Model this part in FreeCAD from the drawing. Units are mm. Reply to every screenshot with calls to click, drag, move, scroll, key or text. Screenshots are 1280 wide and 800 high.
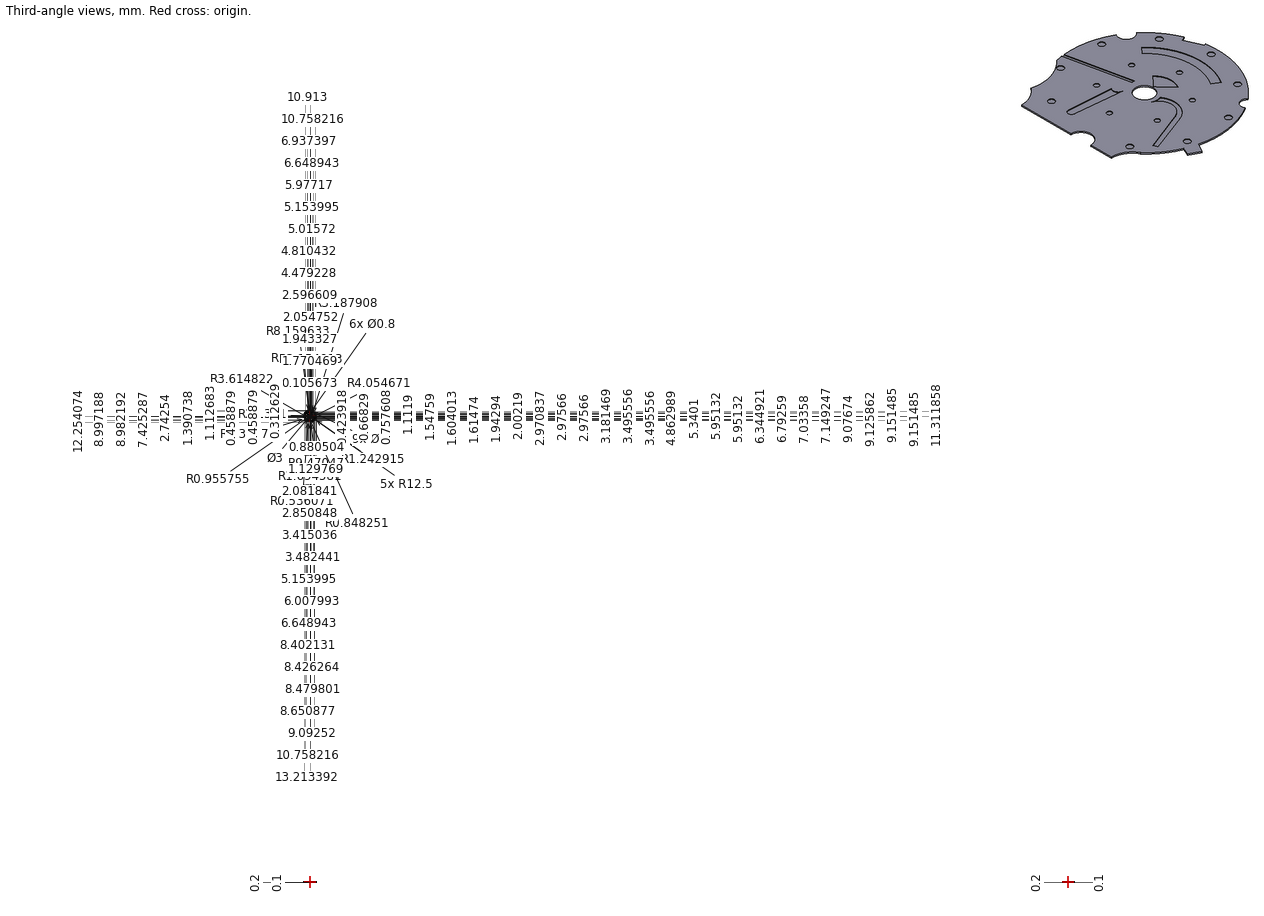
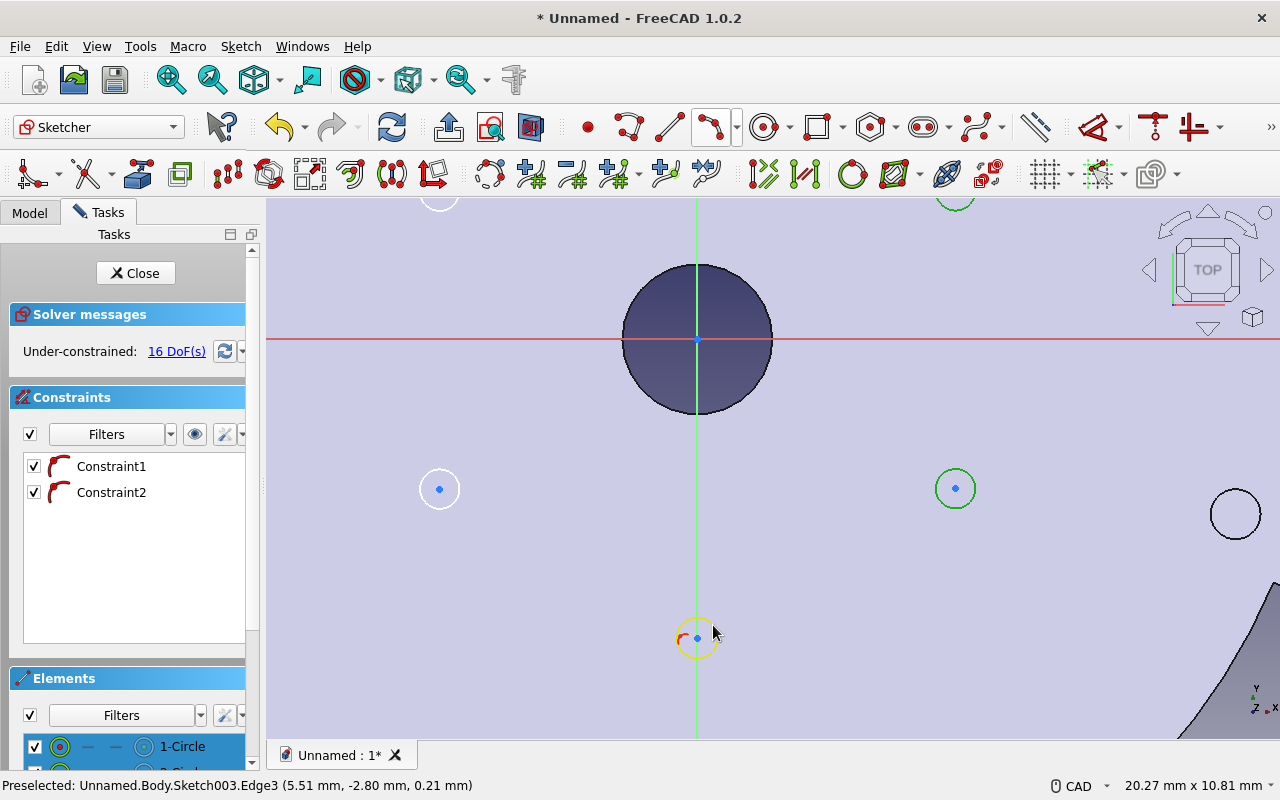
click(712, 624)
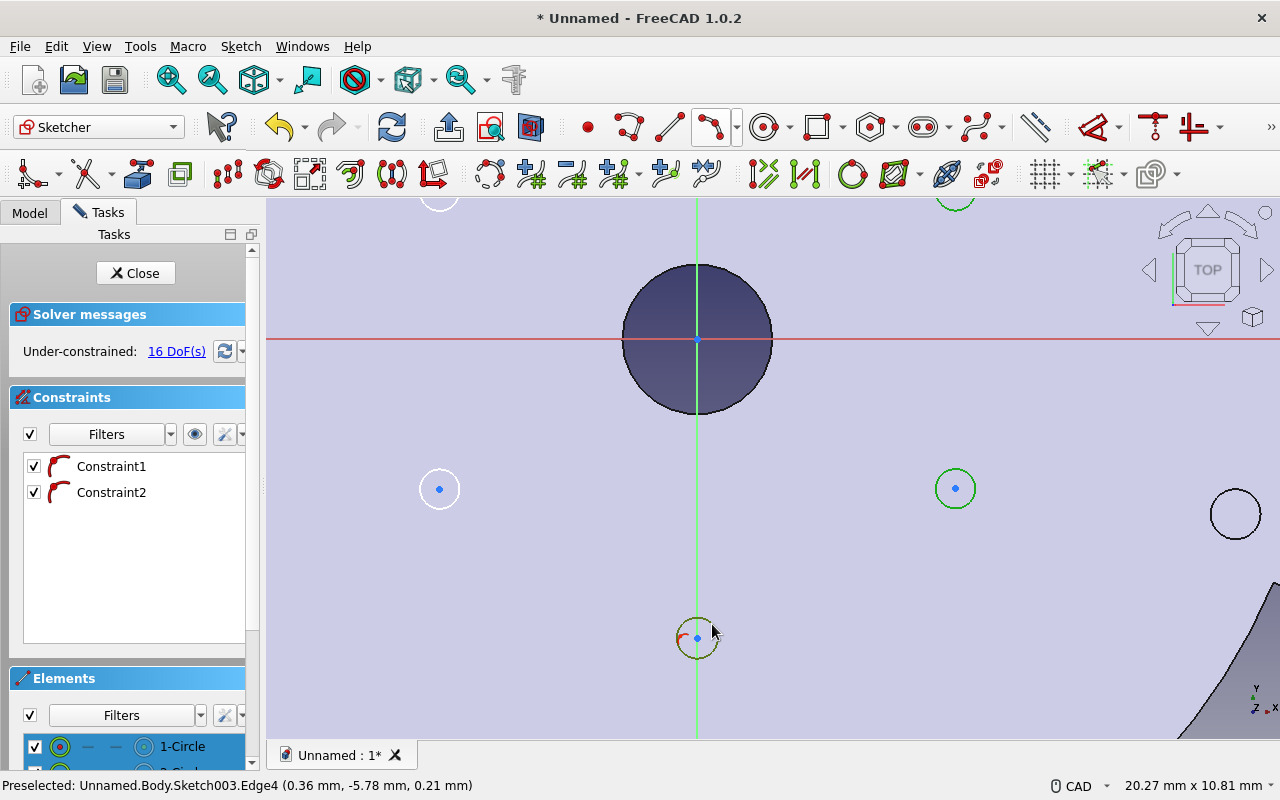
click(454, 475)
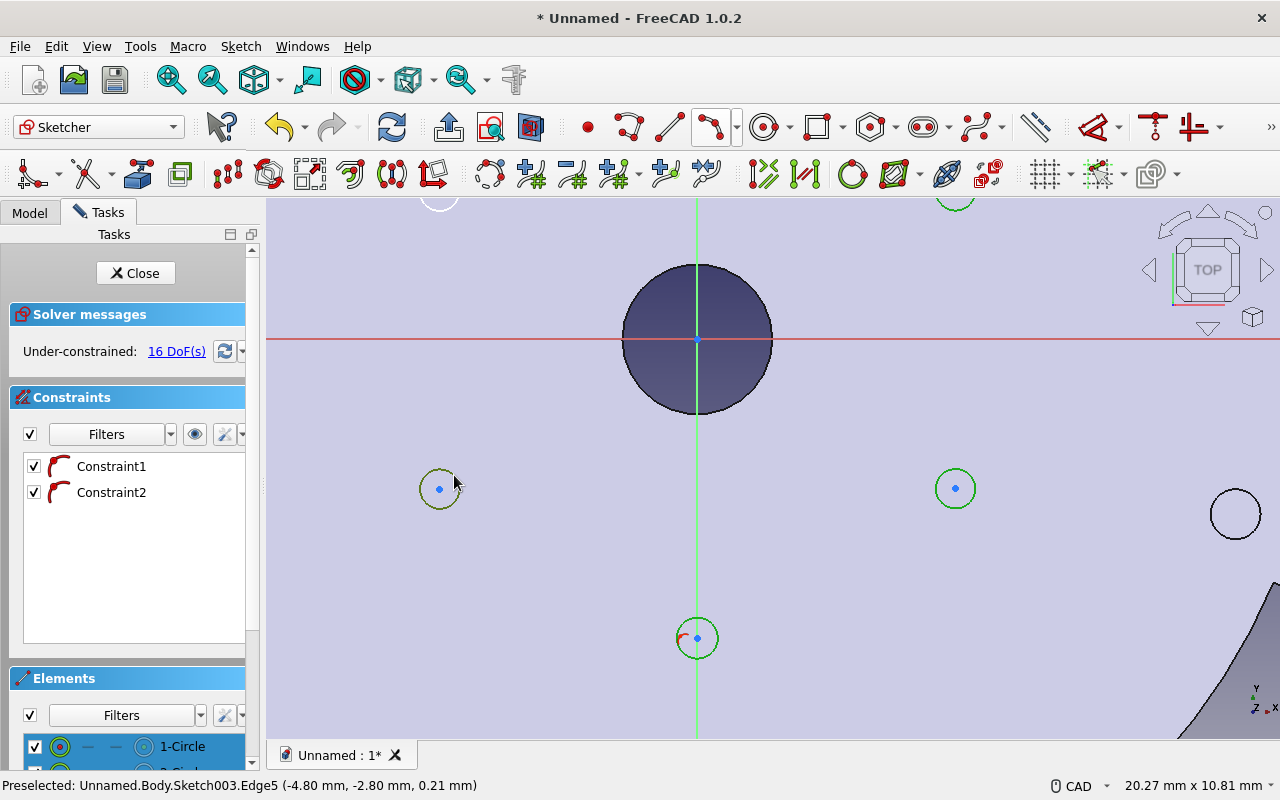
scroll(713, 626, down, 3)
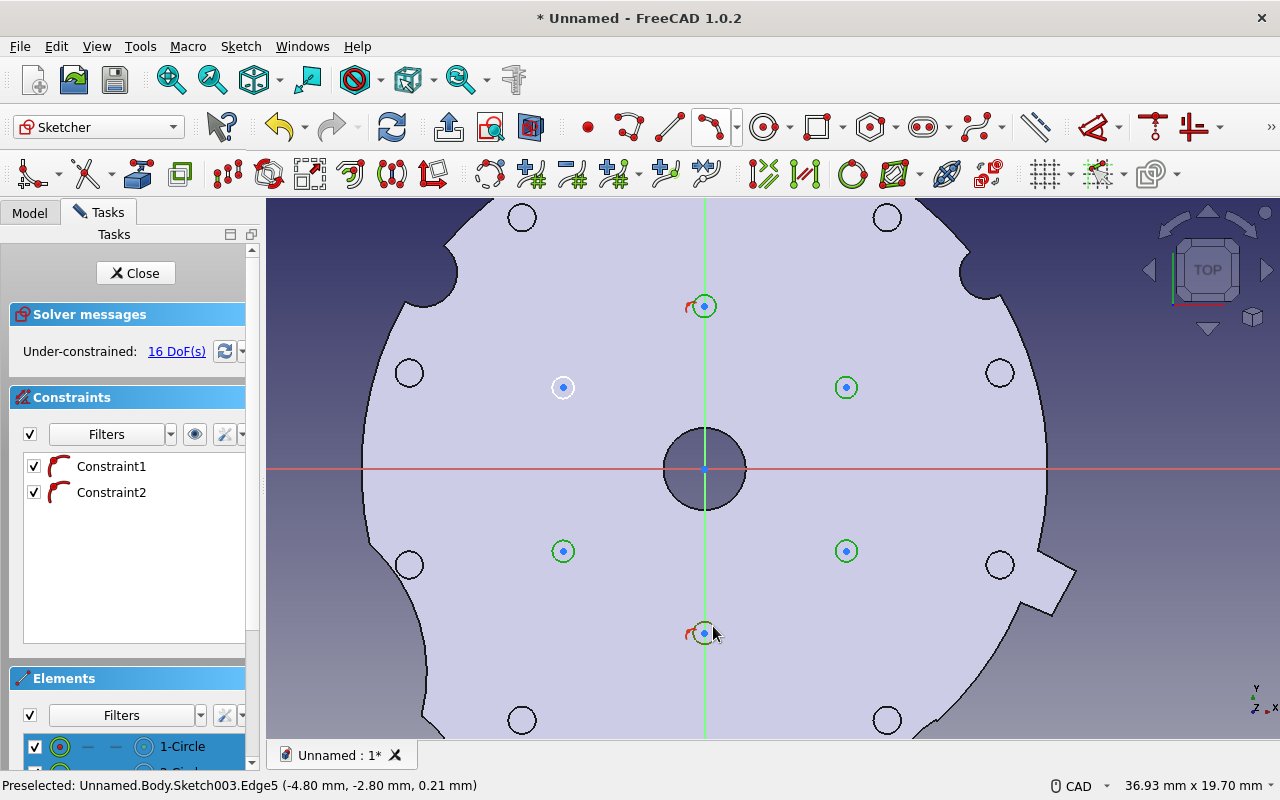
scroll(571, 380, up, 2)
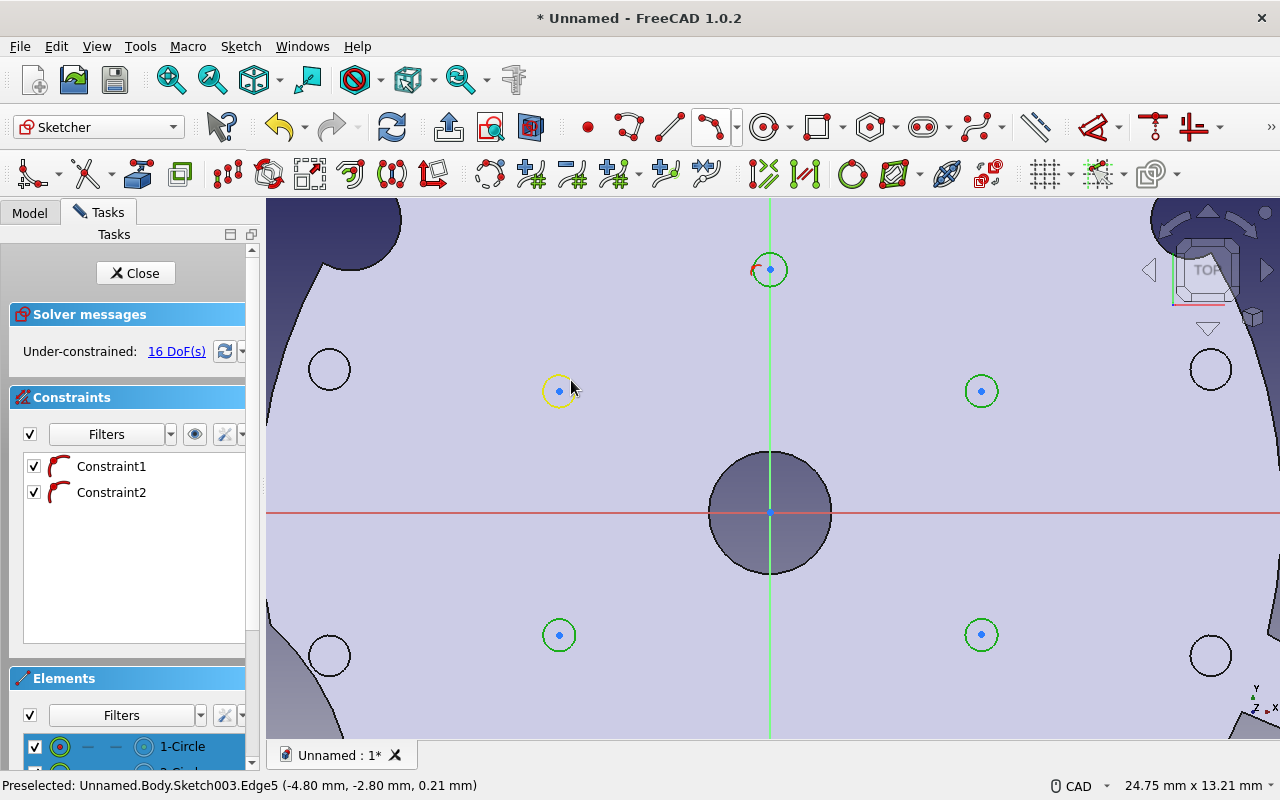
click(571, 380)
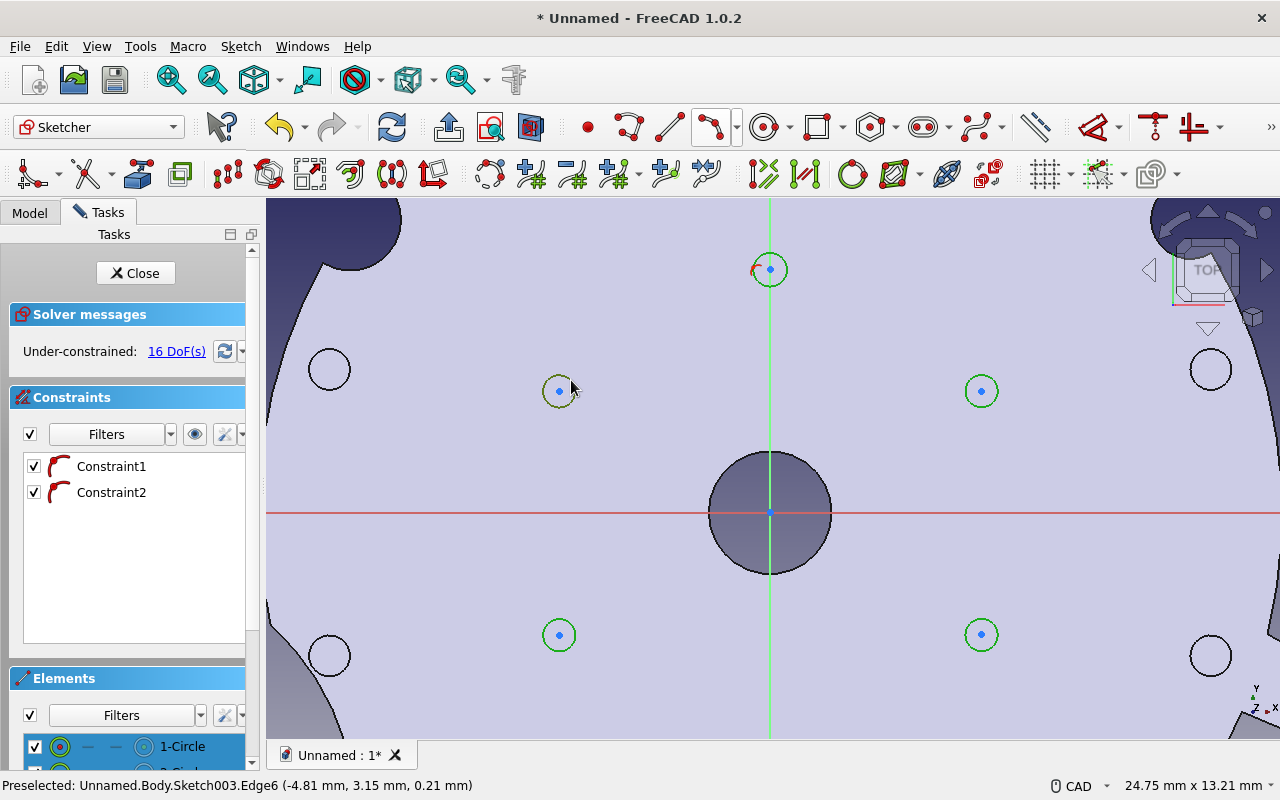
key(e)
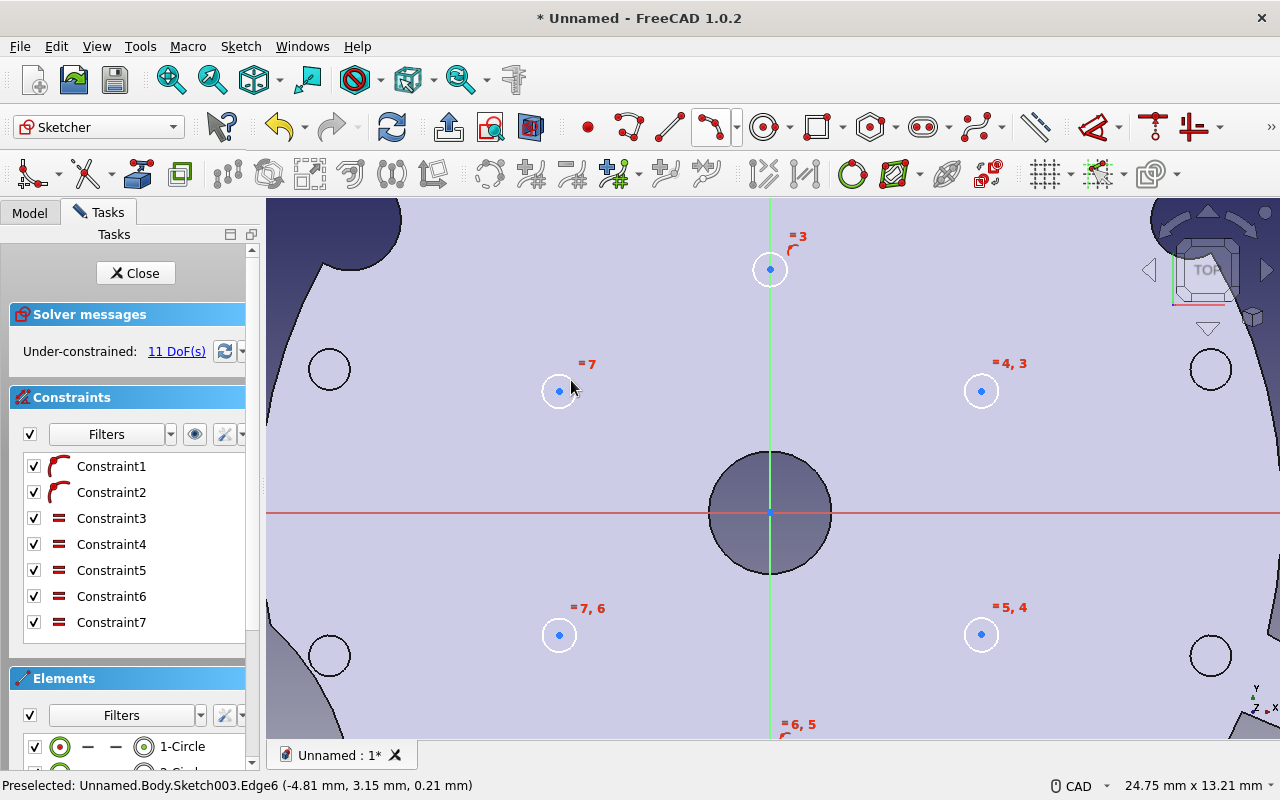
key(d)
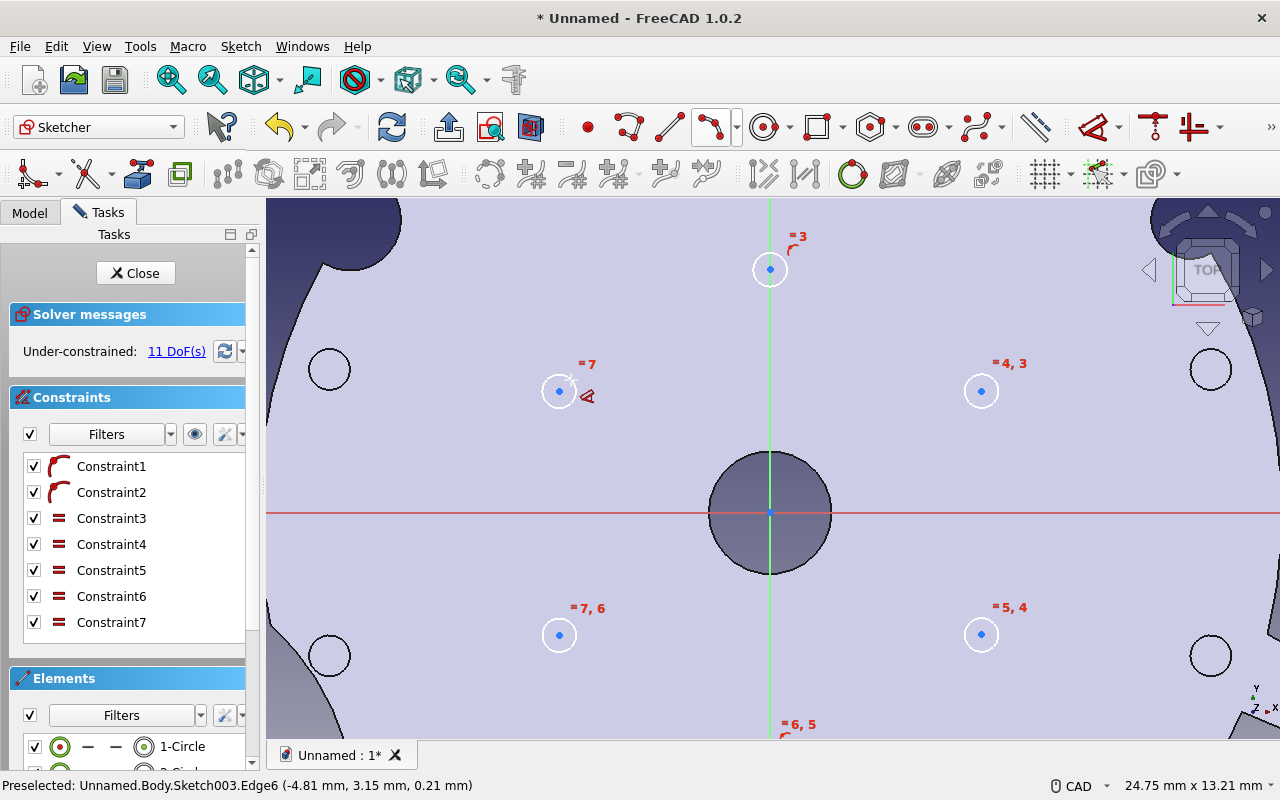
click(782, 258)
click(805, 235)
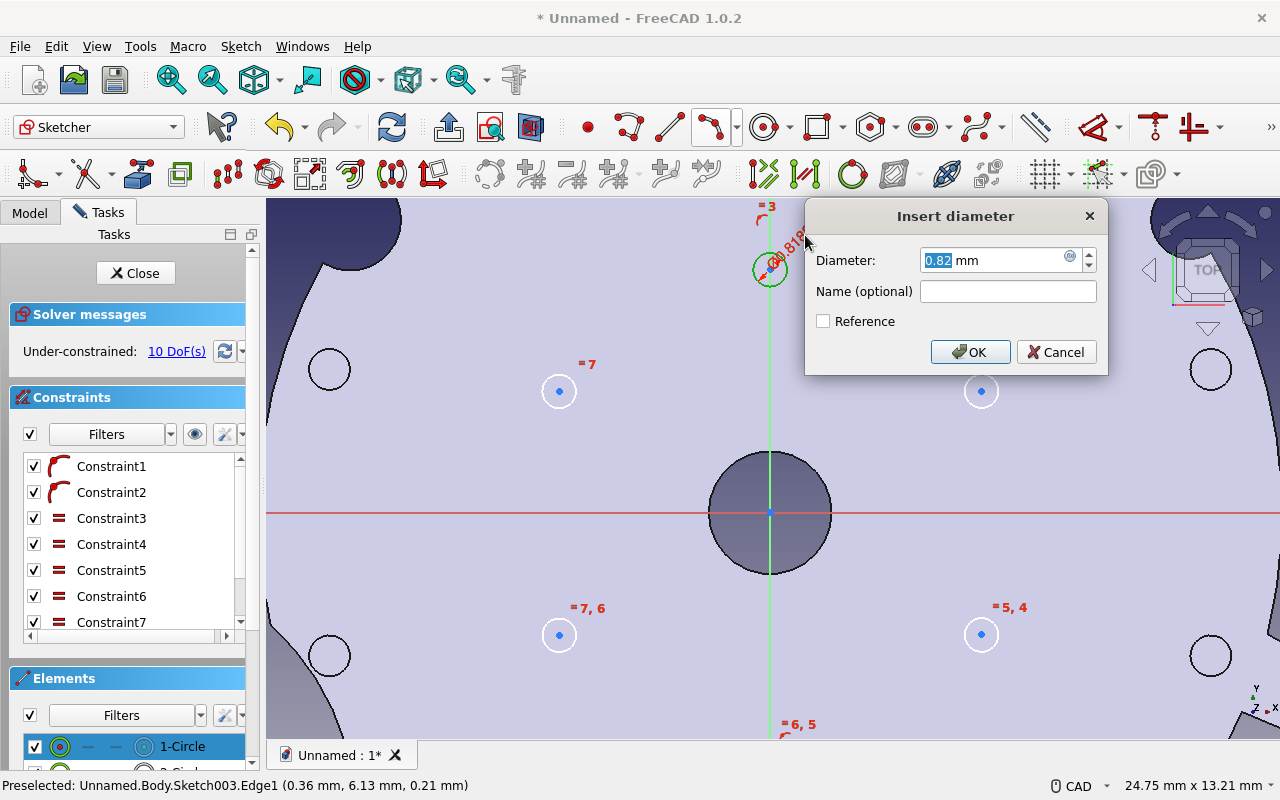
text(0.8)
key(Return)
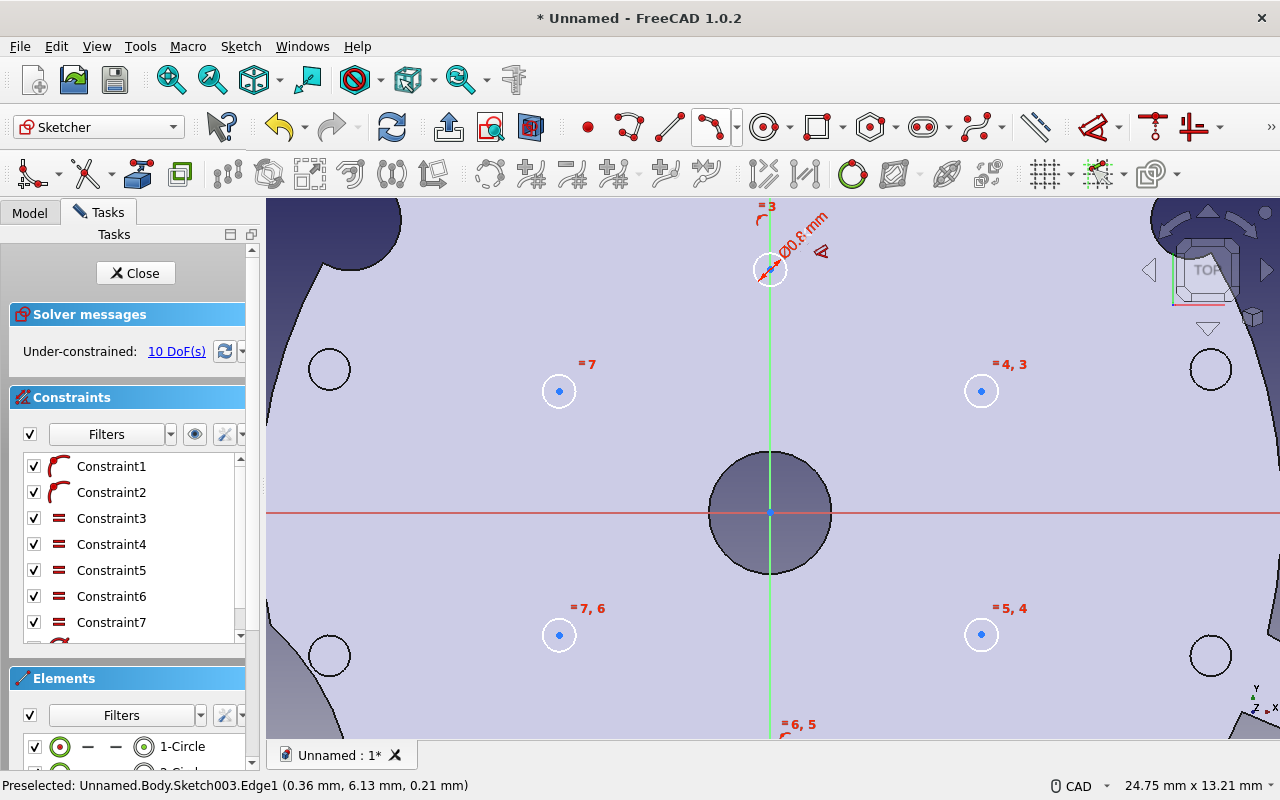
click(770, 270)
click(804, 391)